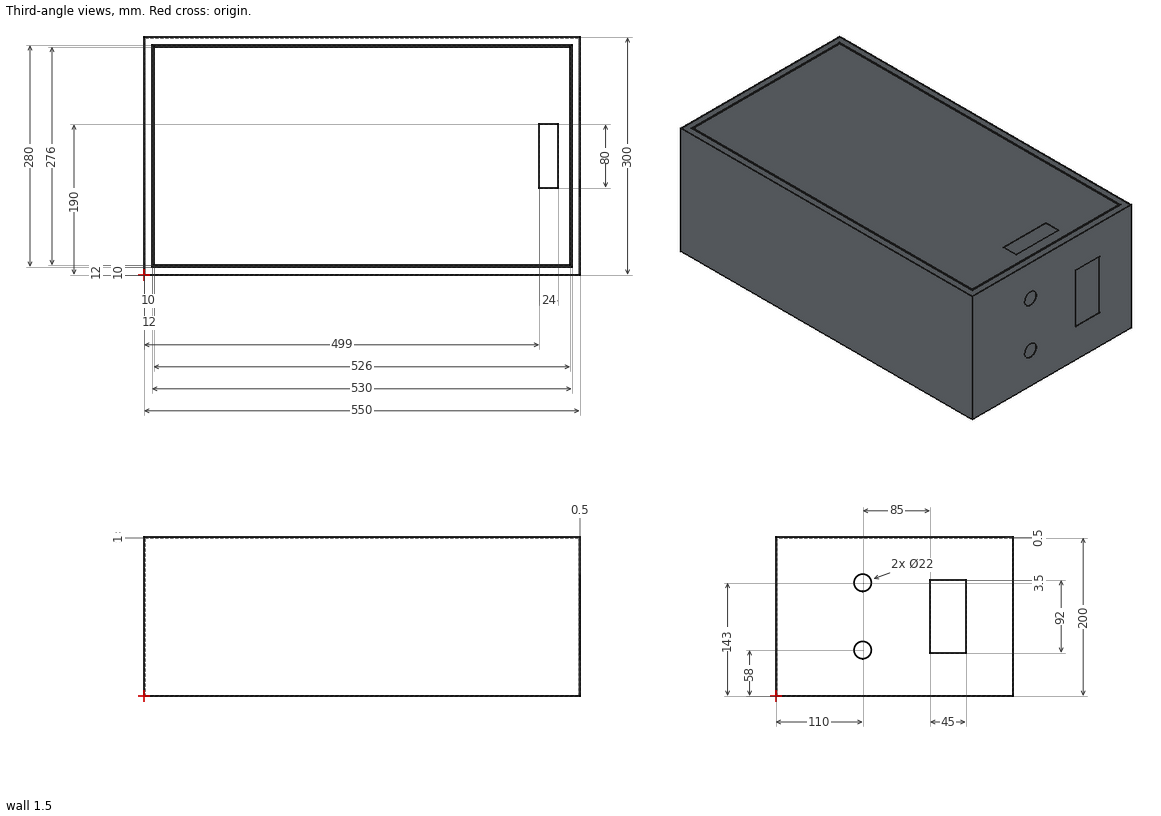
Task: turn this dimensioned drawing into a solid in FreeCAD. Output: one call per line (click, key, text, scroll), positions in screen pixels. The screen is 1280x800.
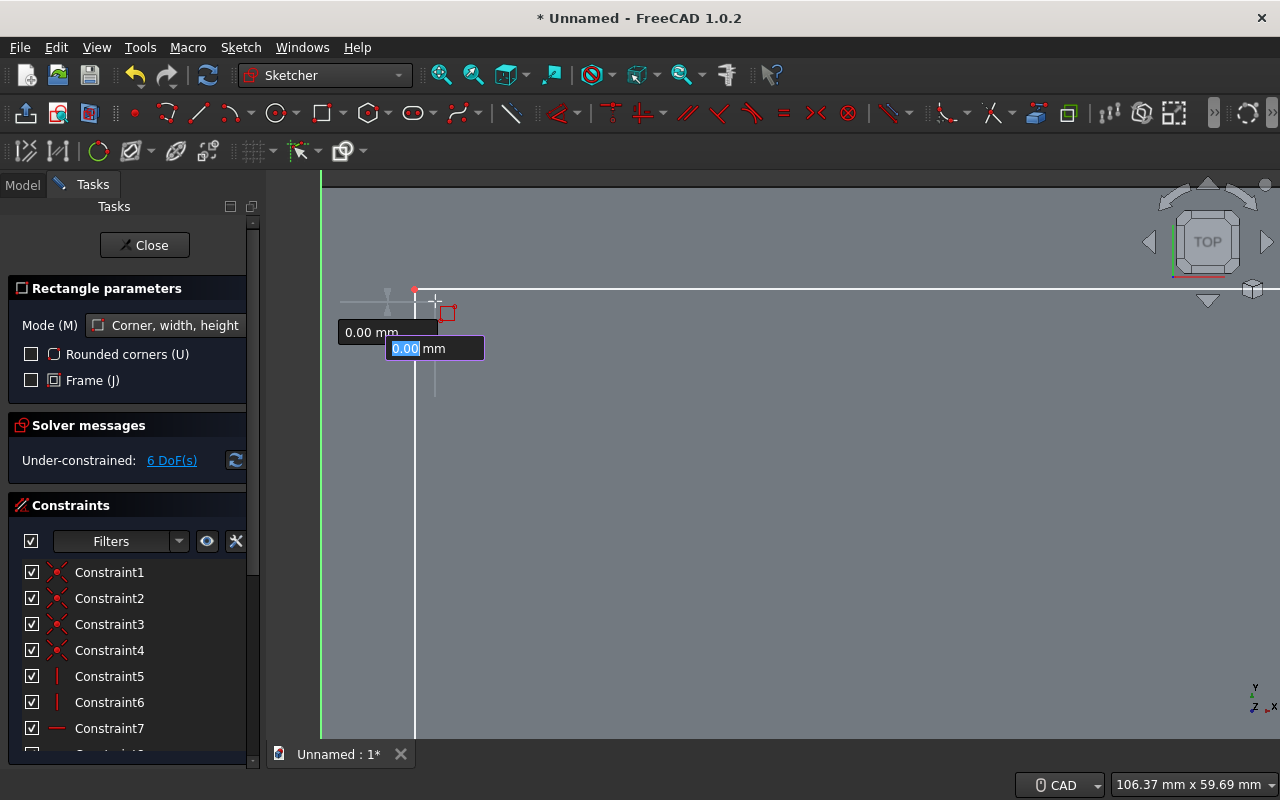
scroll(432, 304, down, 11)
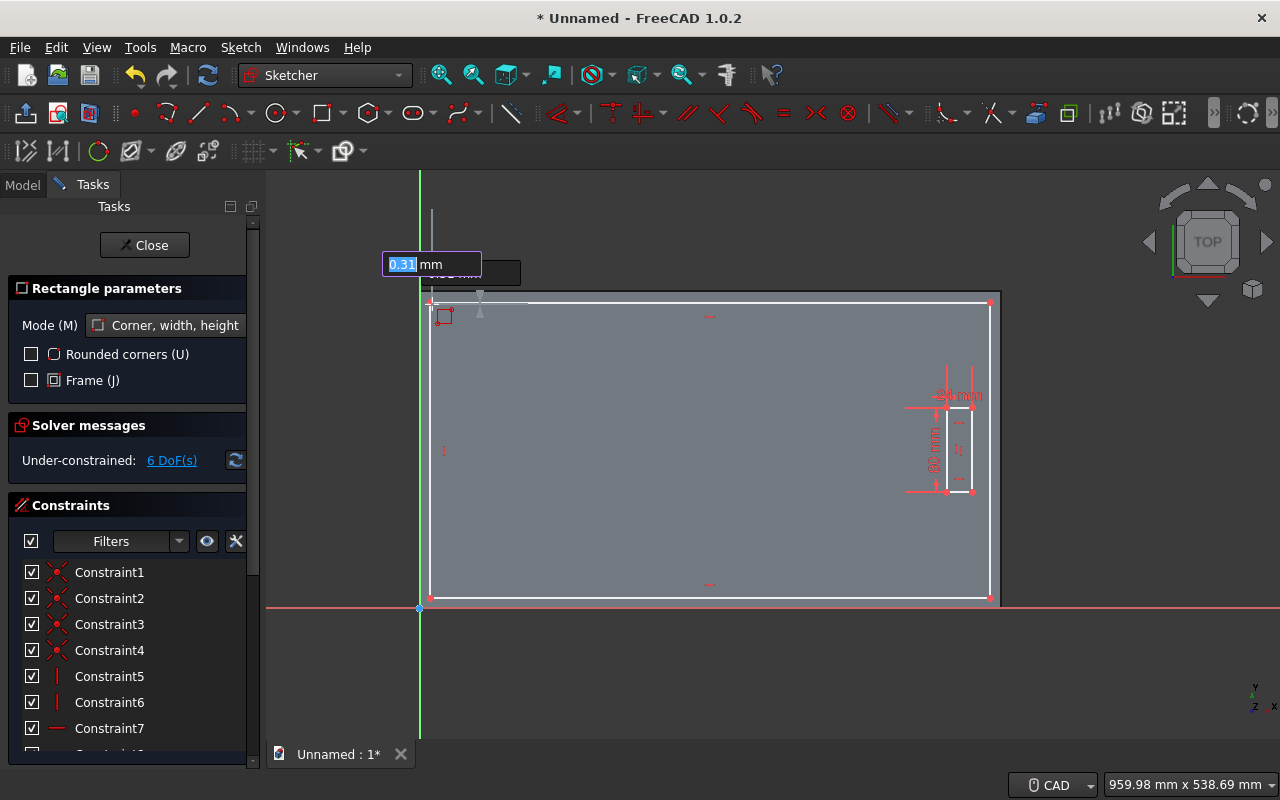
scroll(988, 595, up, 11)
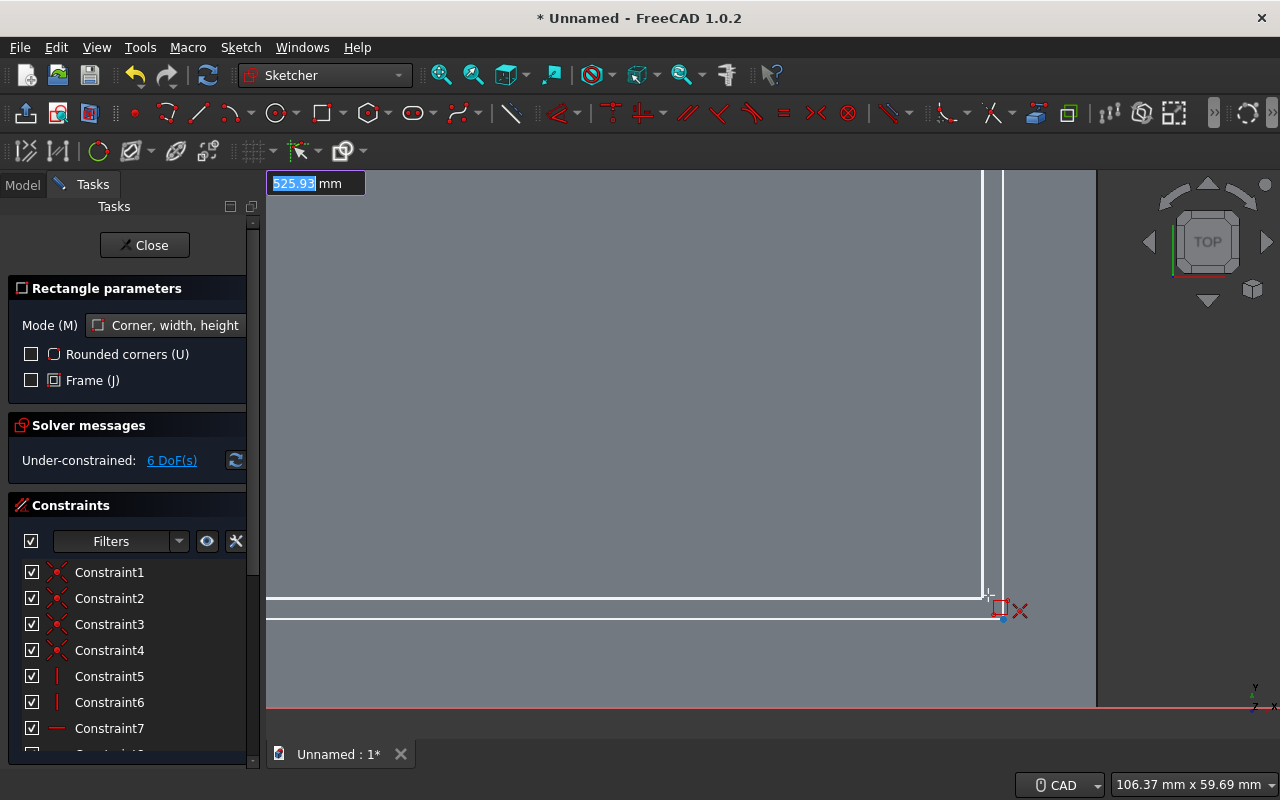
click(983, 593)
key(Escape)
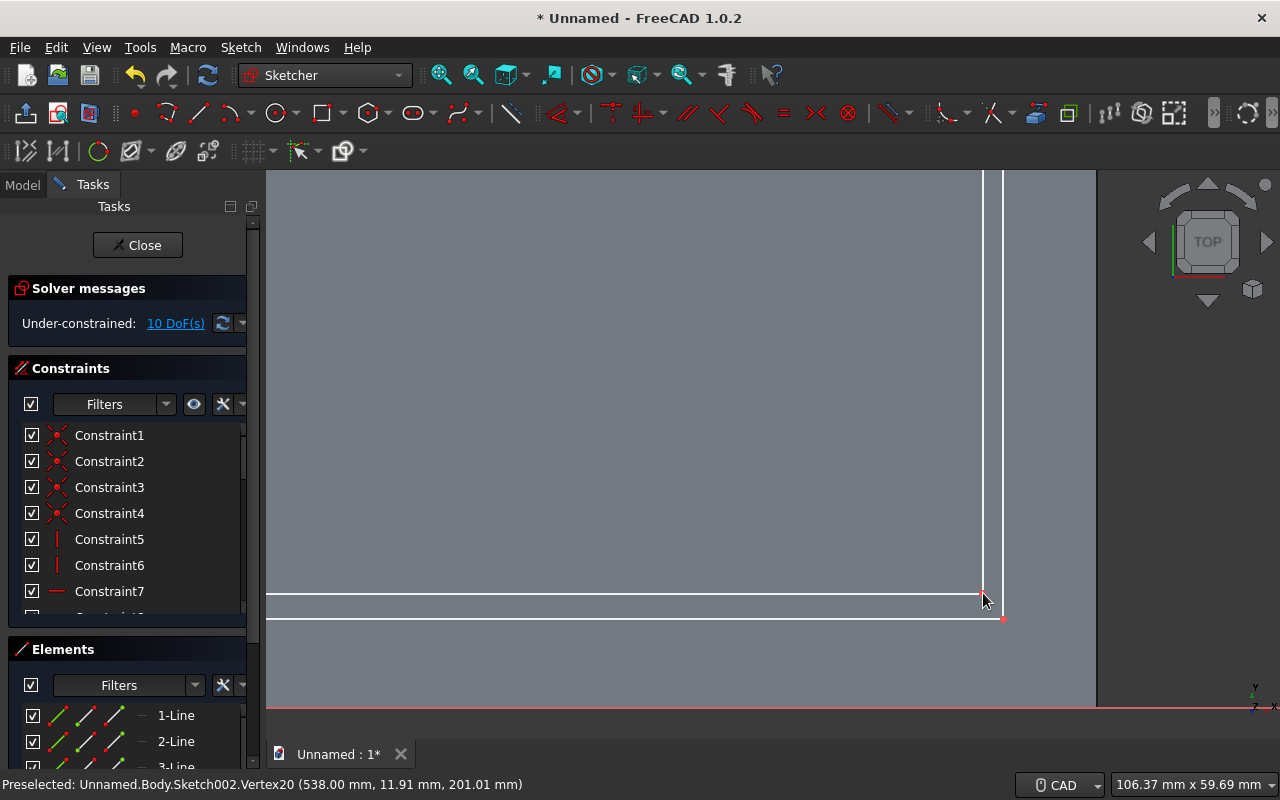
click(558, 114)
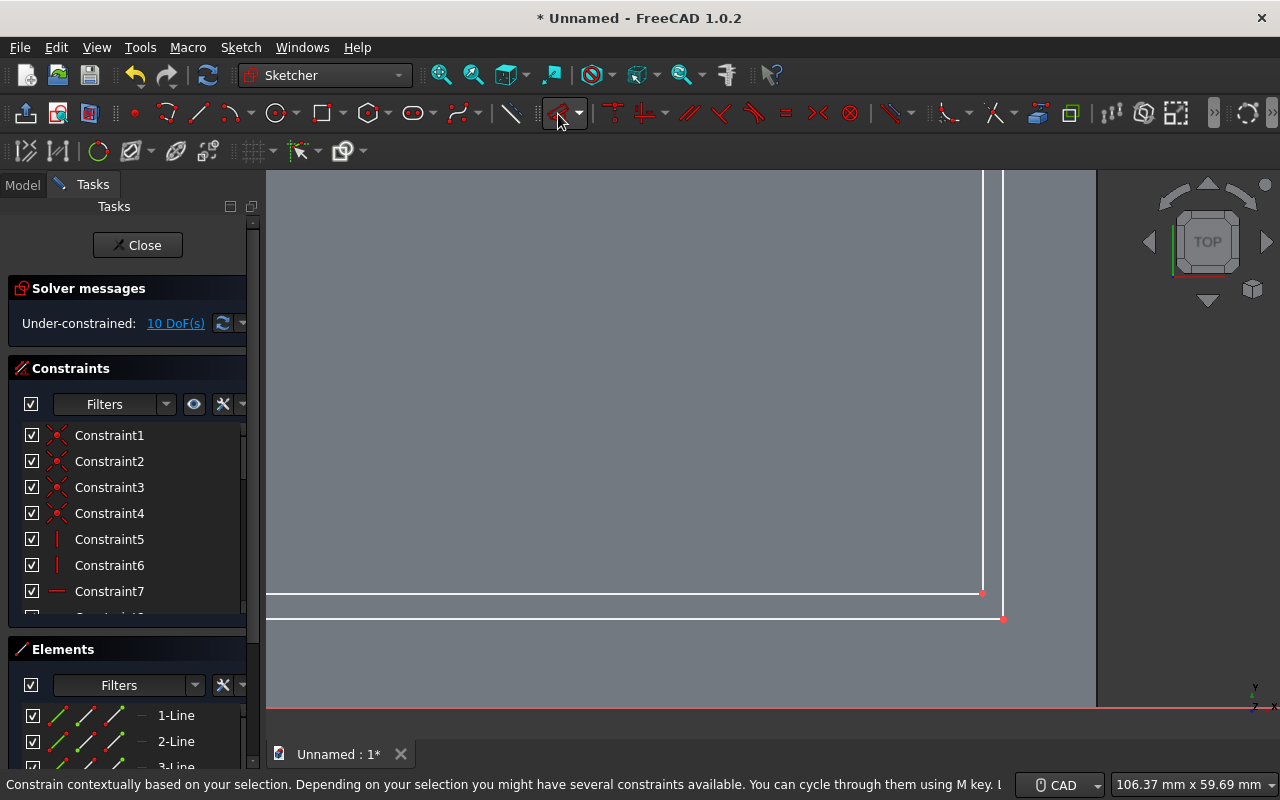
scroll(988, 595, down, 11)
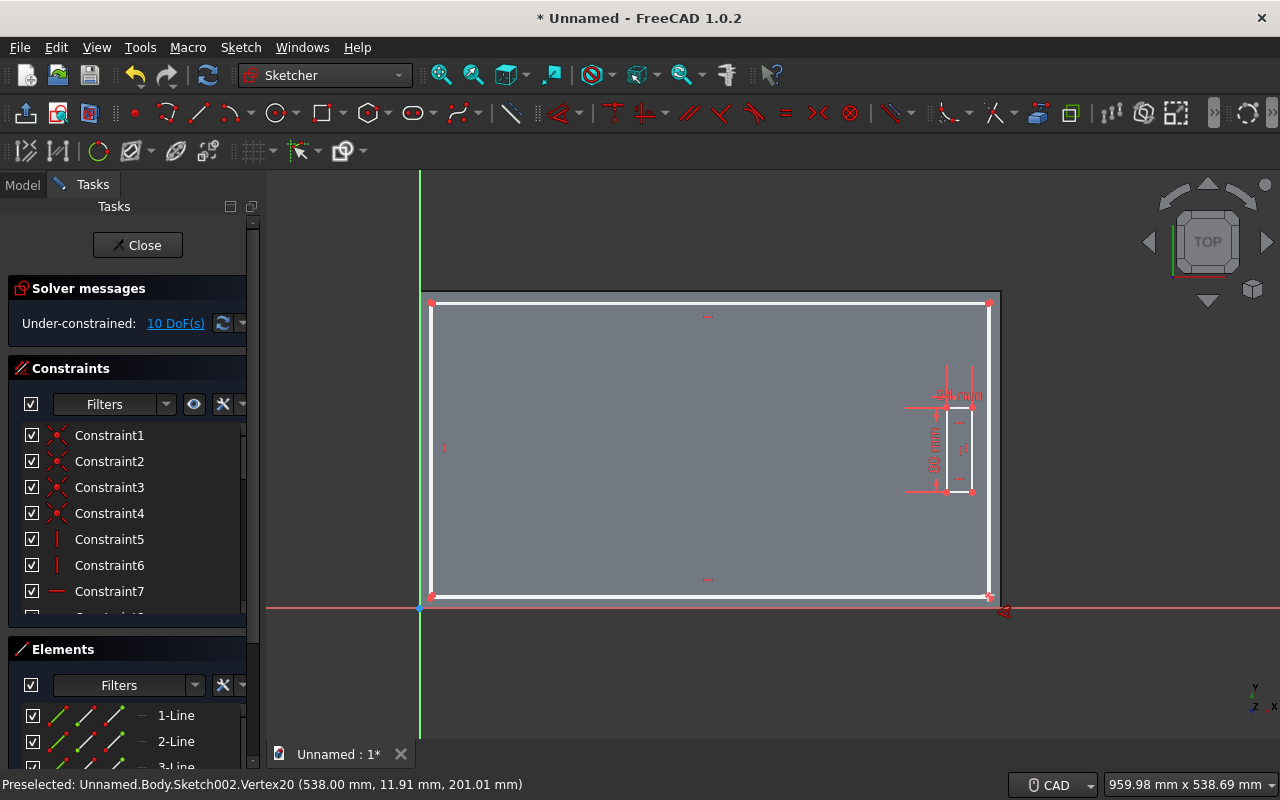
scroll(430, 391, up, 10)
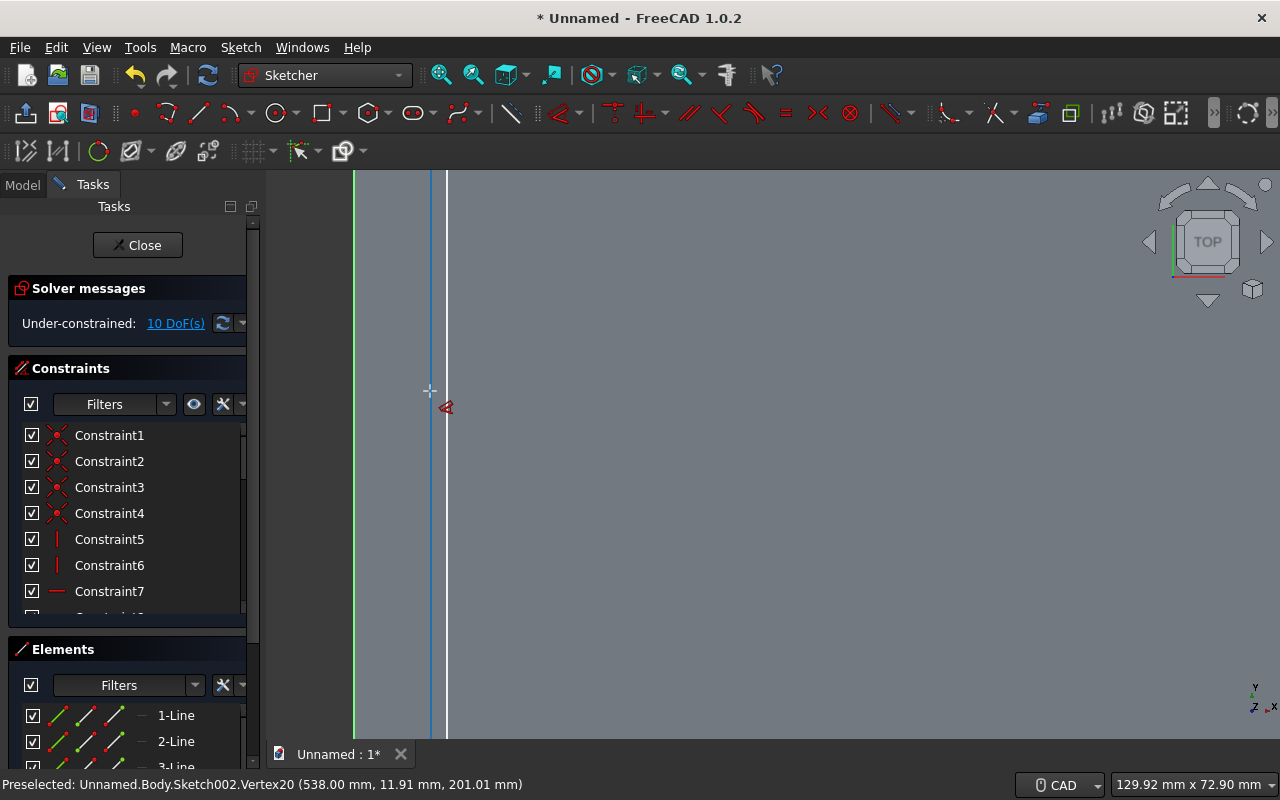
click(431, 391)
click(397, 454)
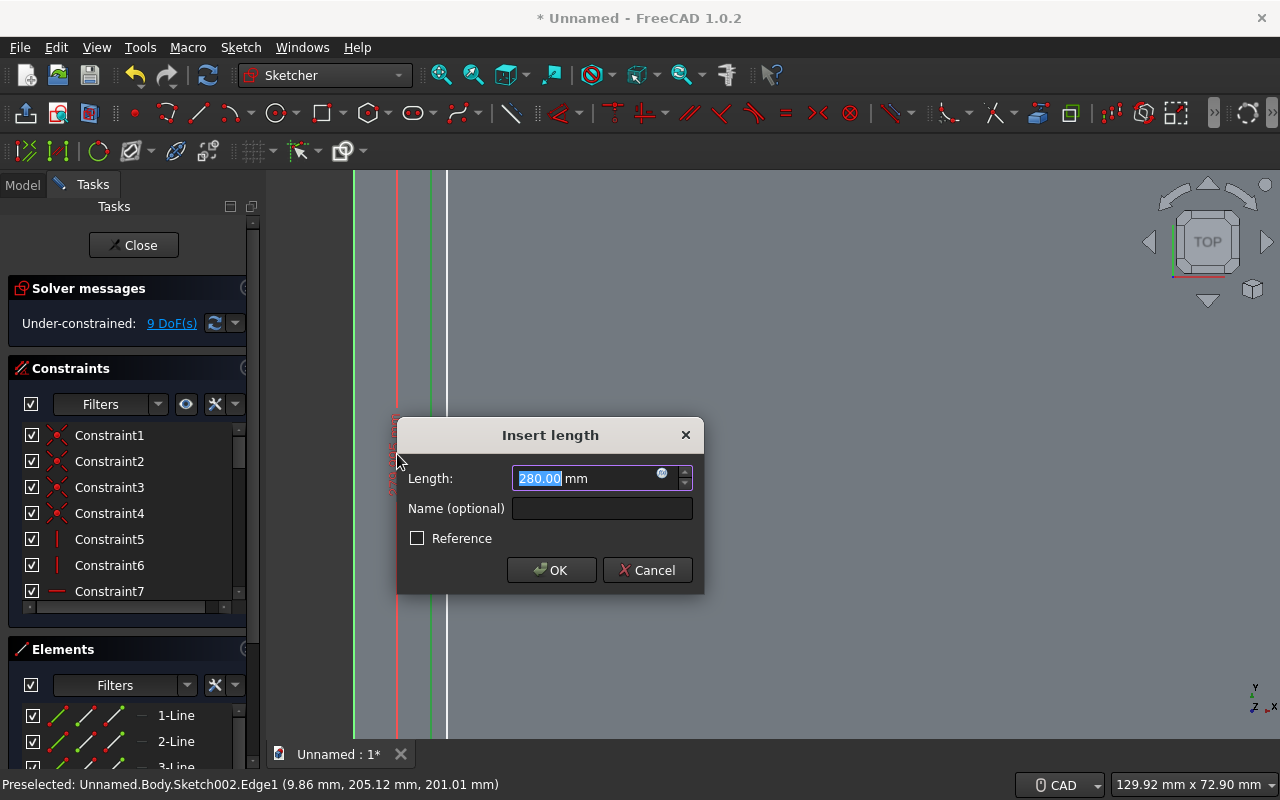
text(280)
key(Return)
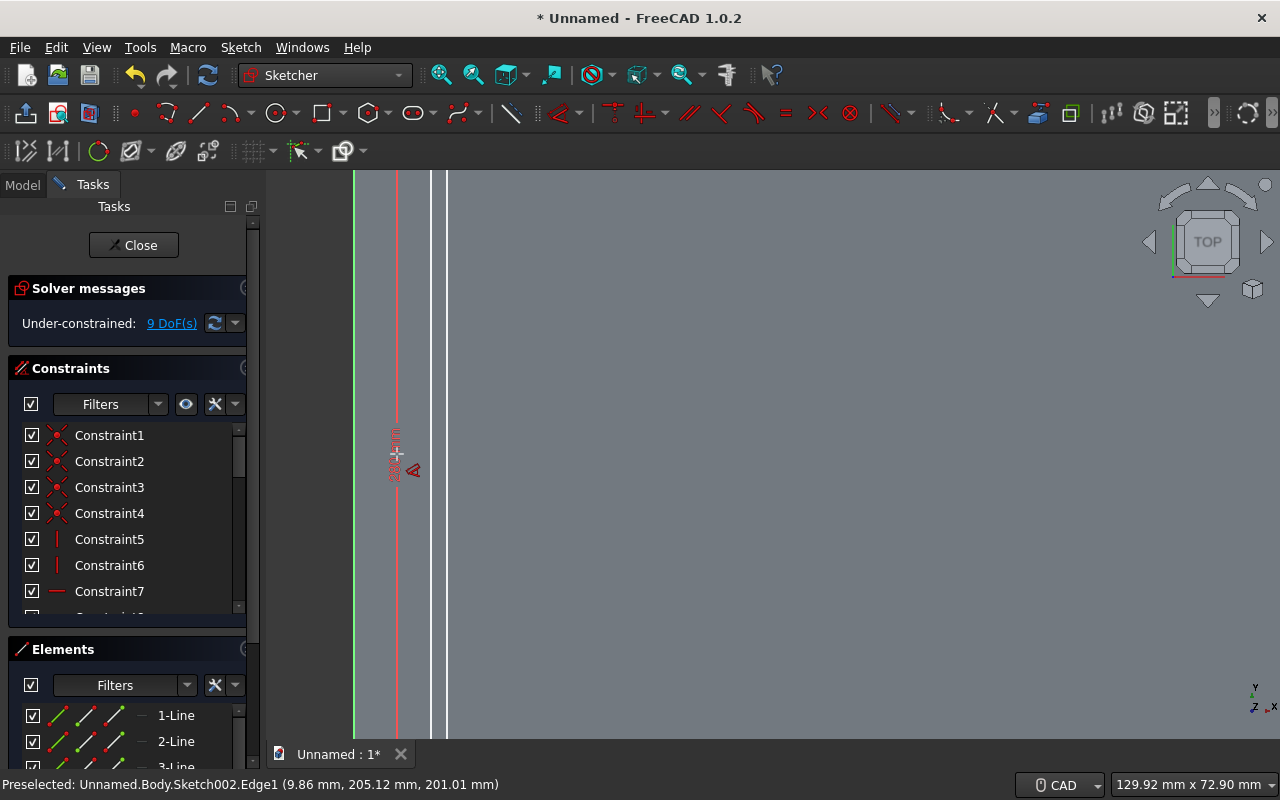
scroll(430, 391, down, 10)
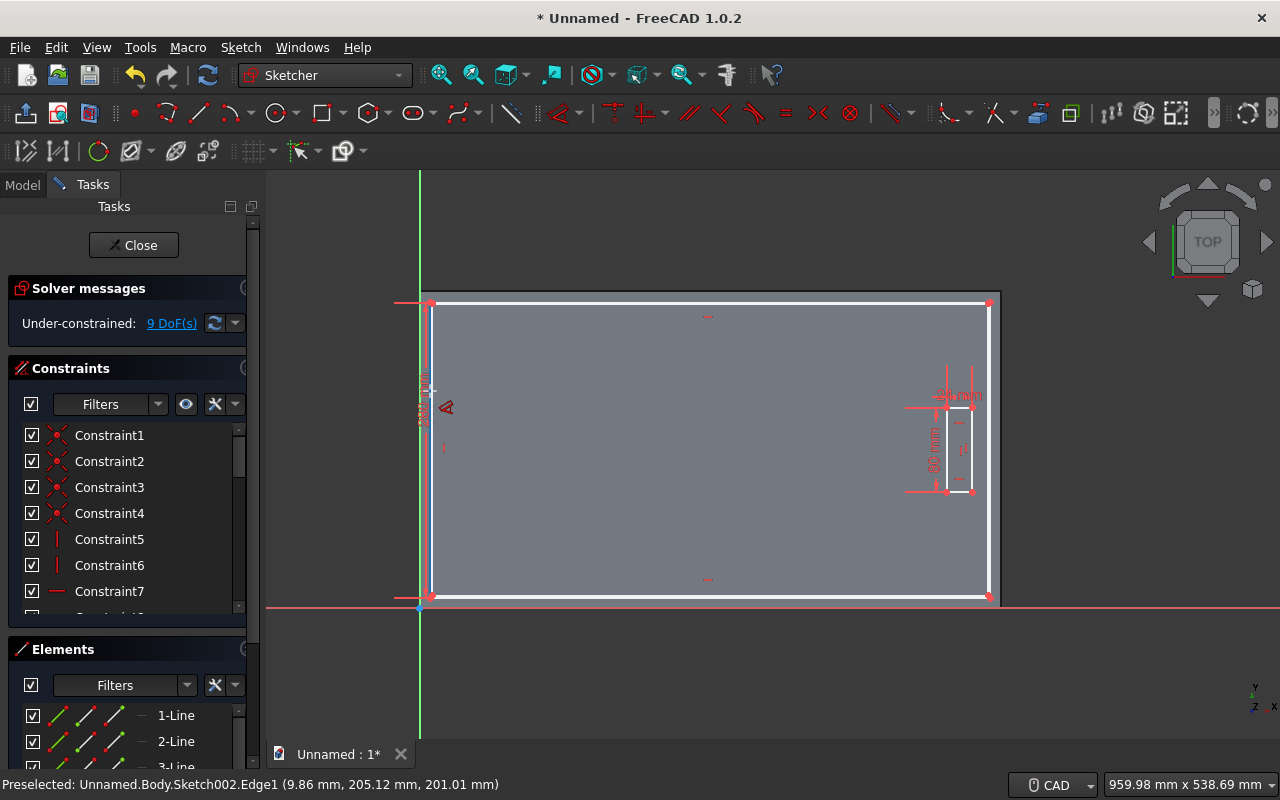
scroll(598, 598, up, 8)